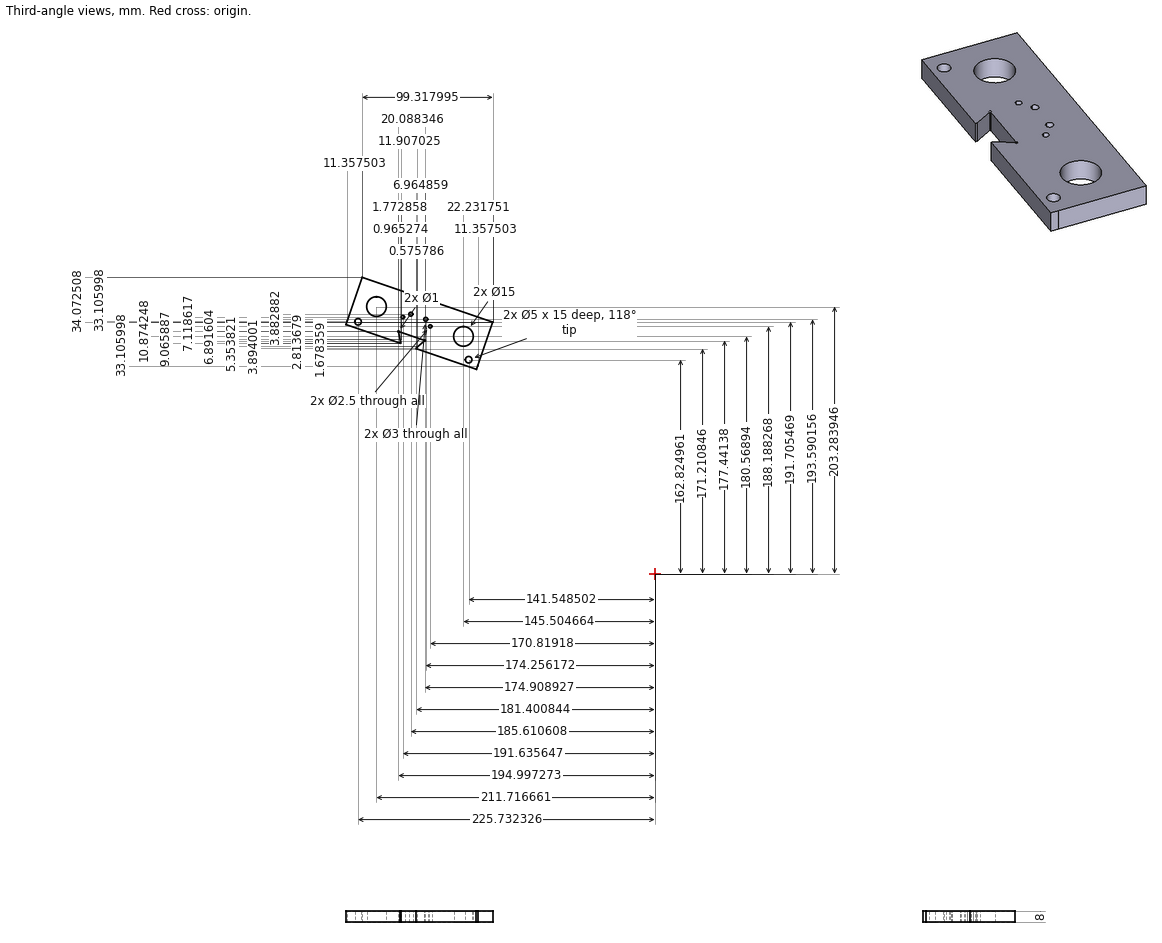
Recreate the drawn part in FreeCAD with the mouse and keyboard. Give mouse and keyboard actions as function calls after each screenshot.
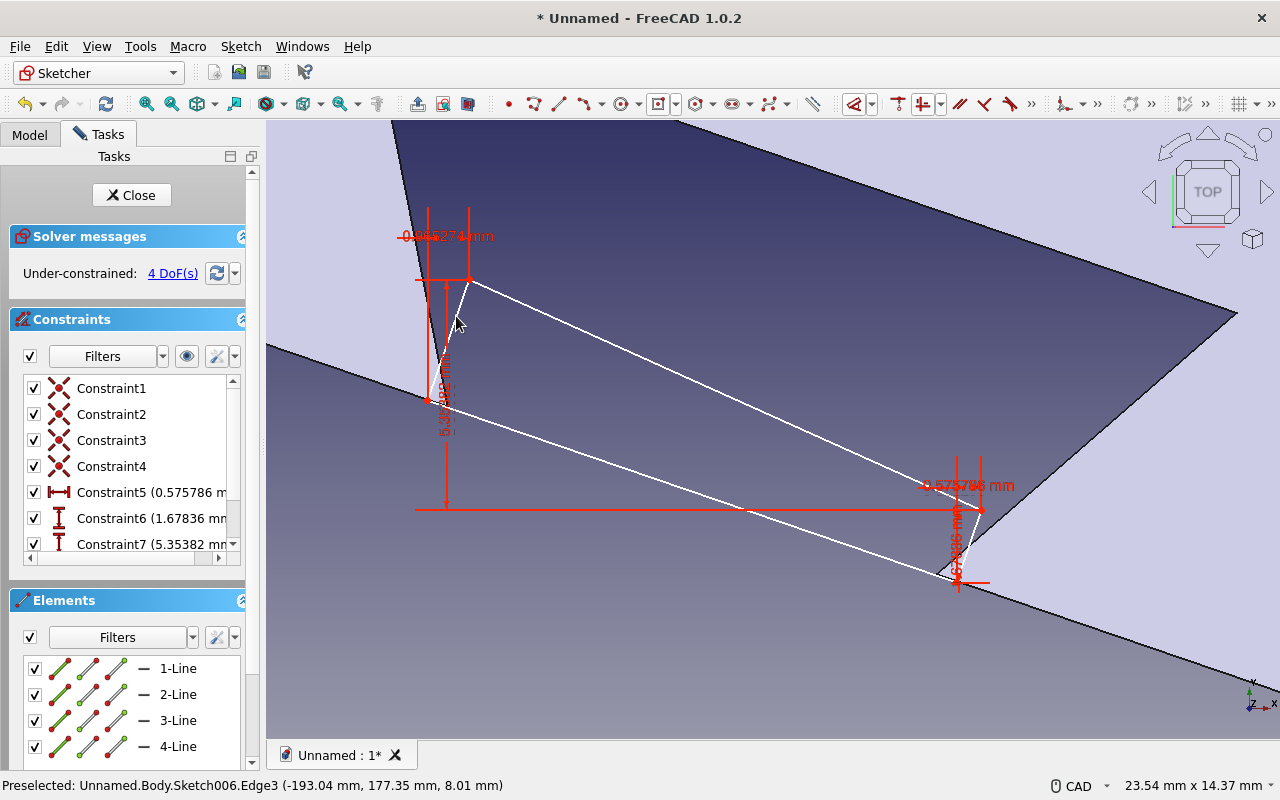
click(457, 316)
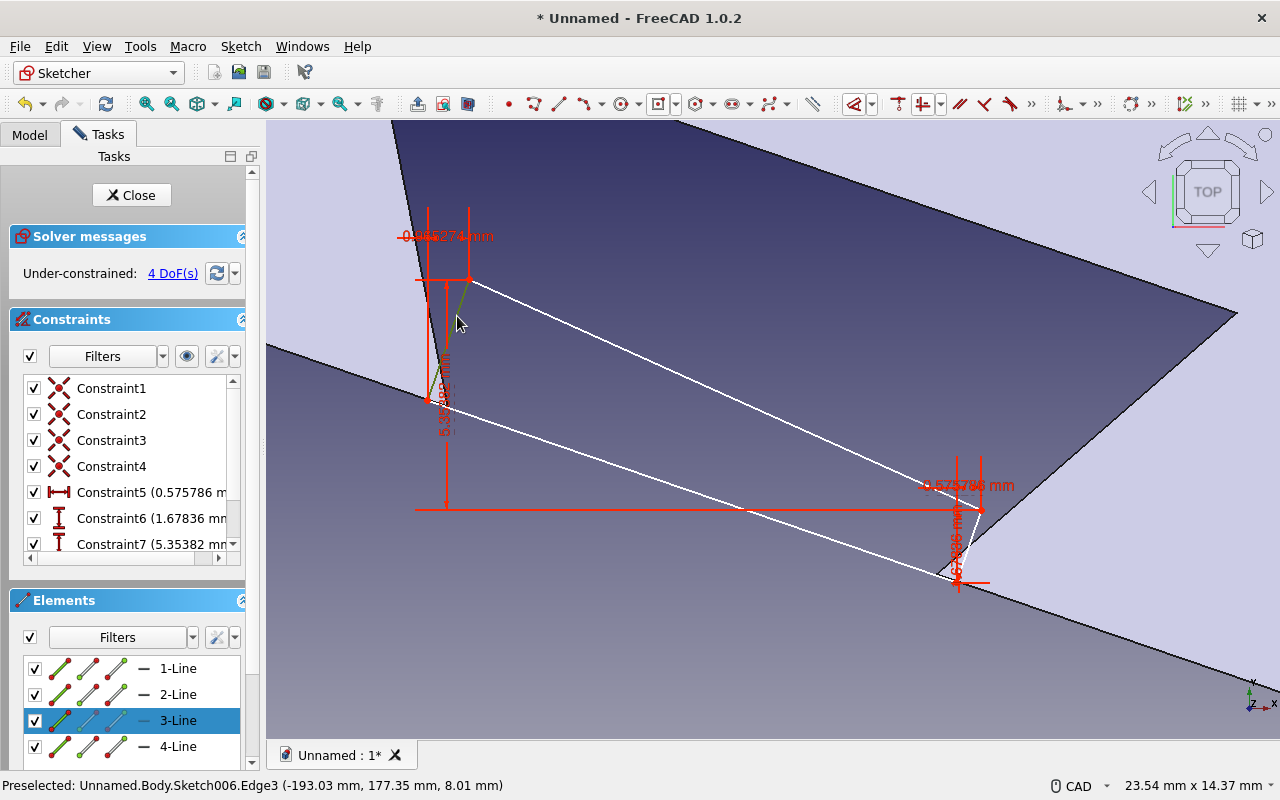
click(872, 104)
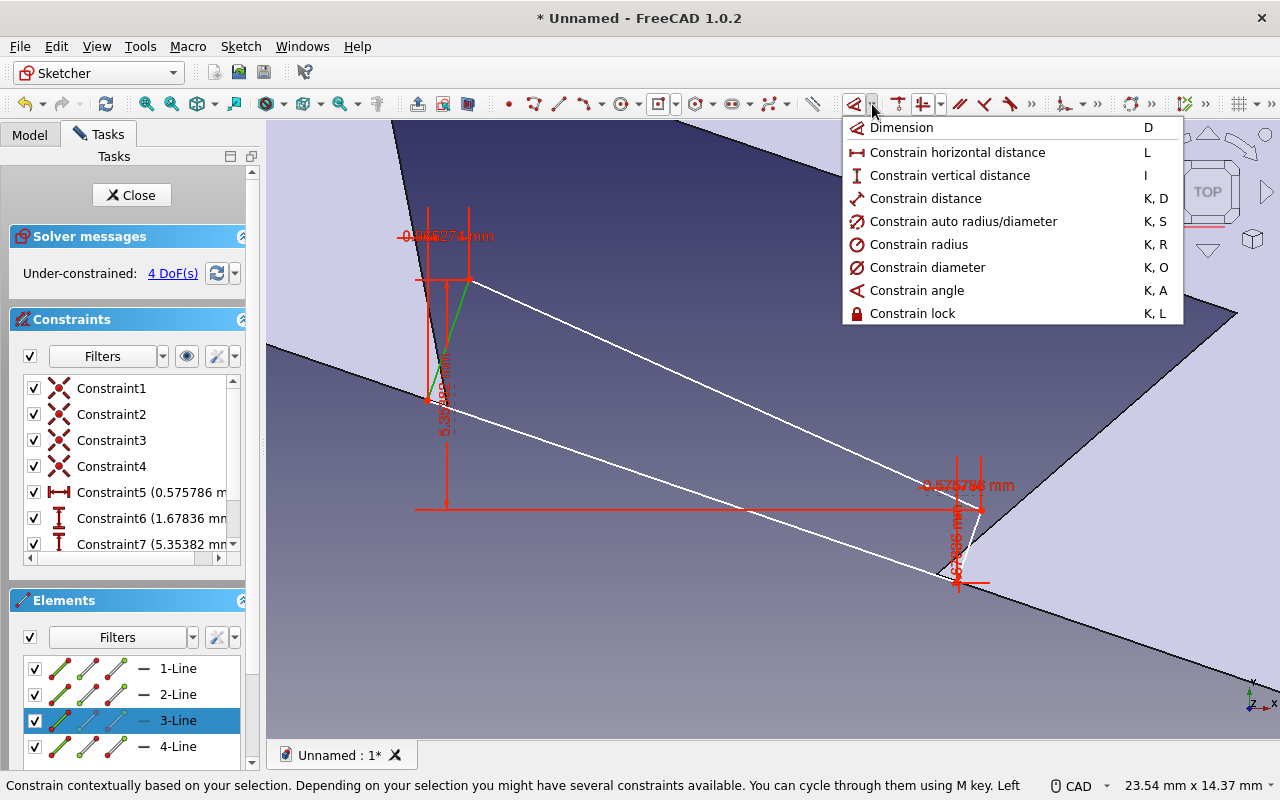
click(1013, 176)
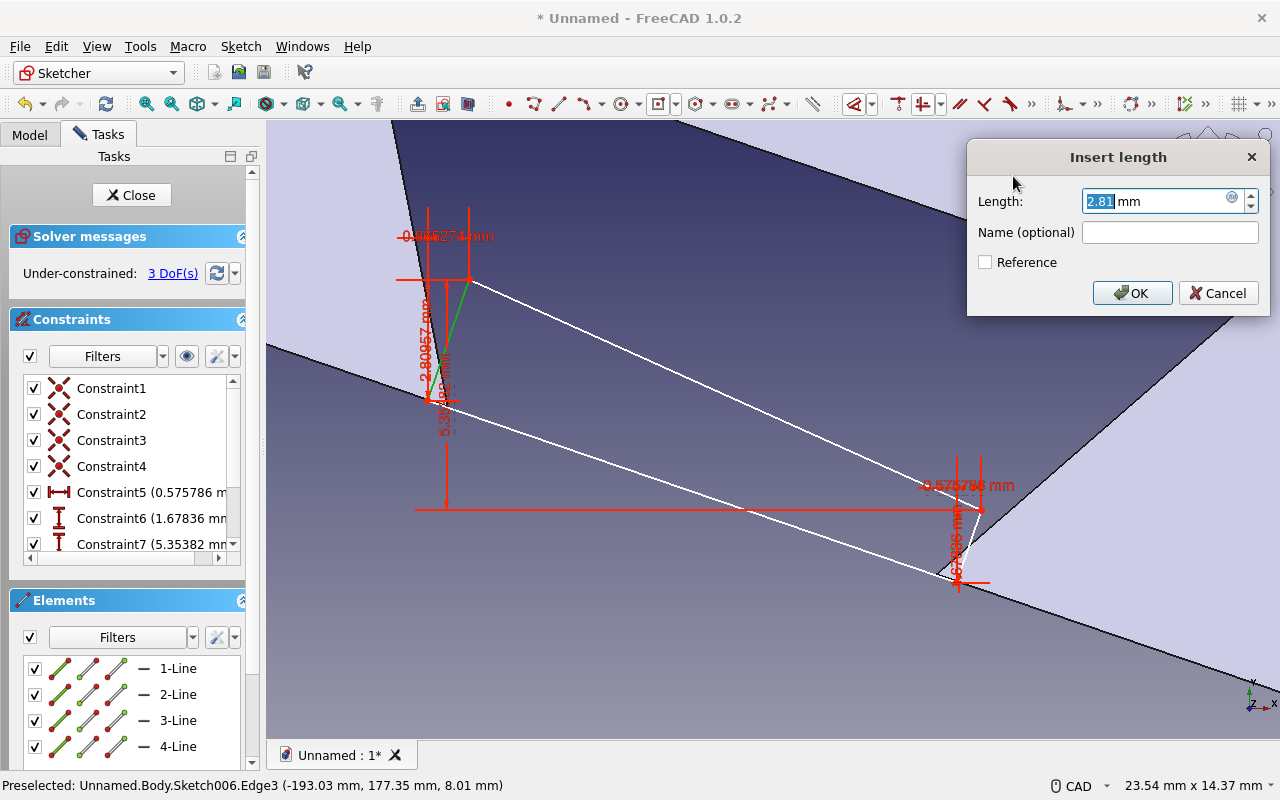
text(2.813679)
key(Return)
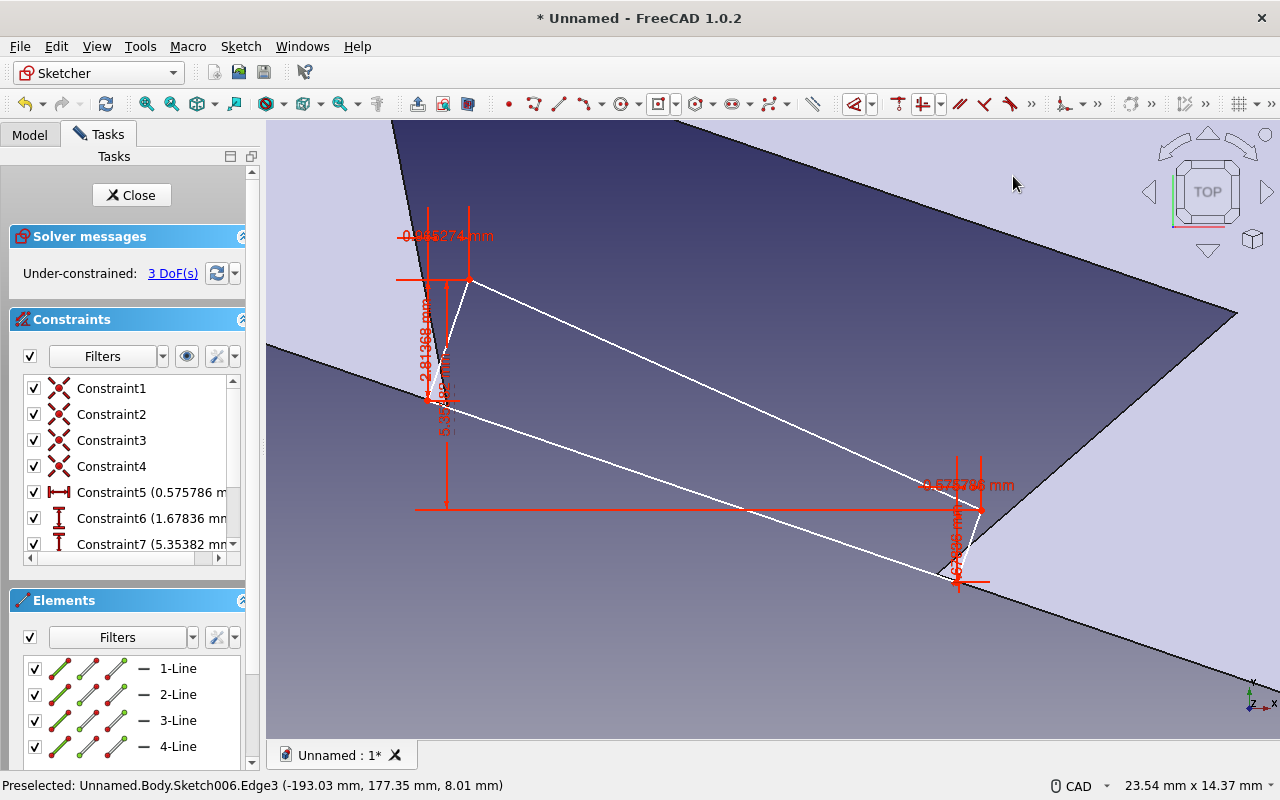
click(828, 441)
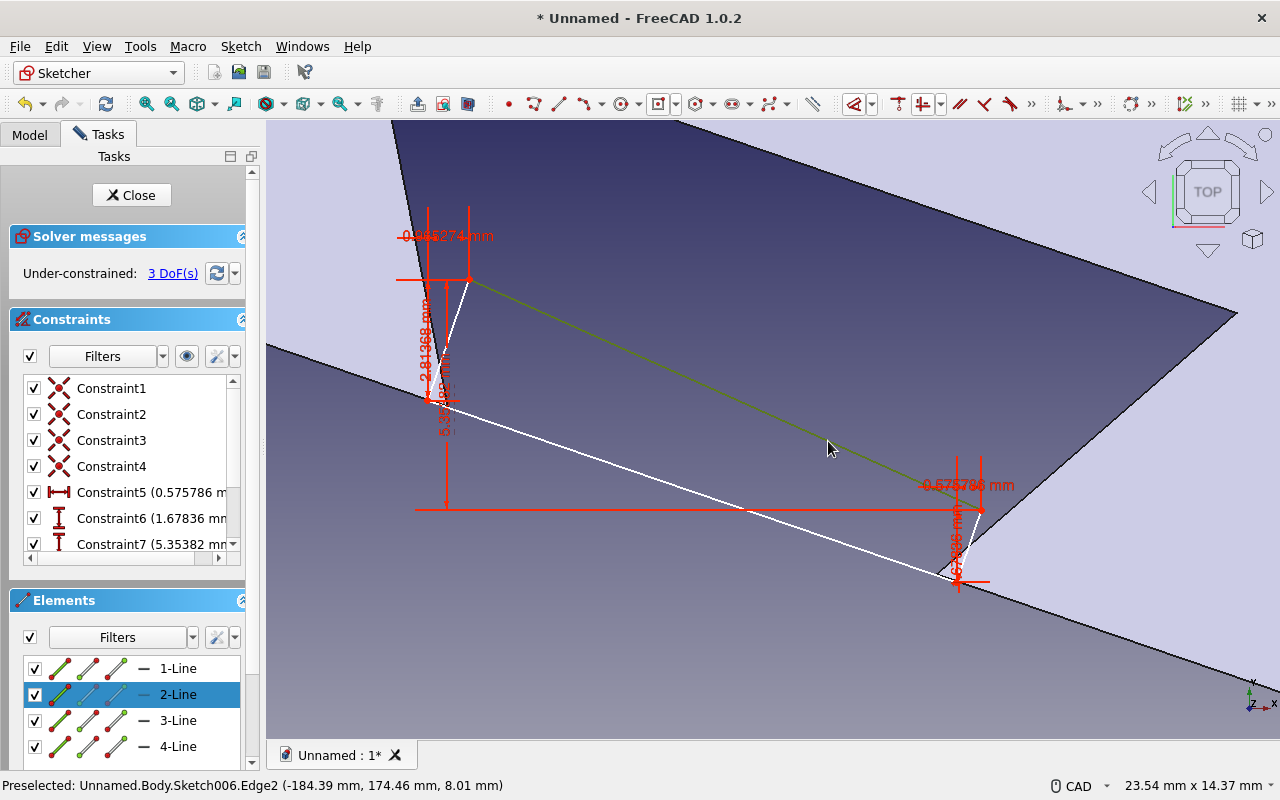
click(872, 104)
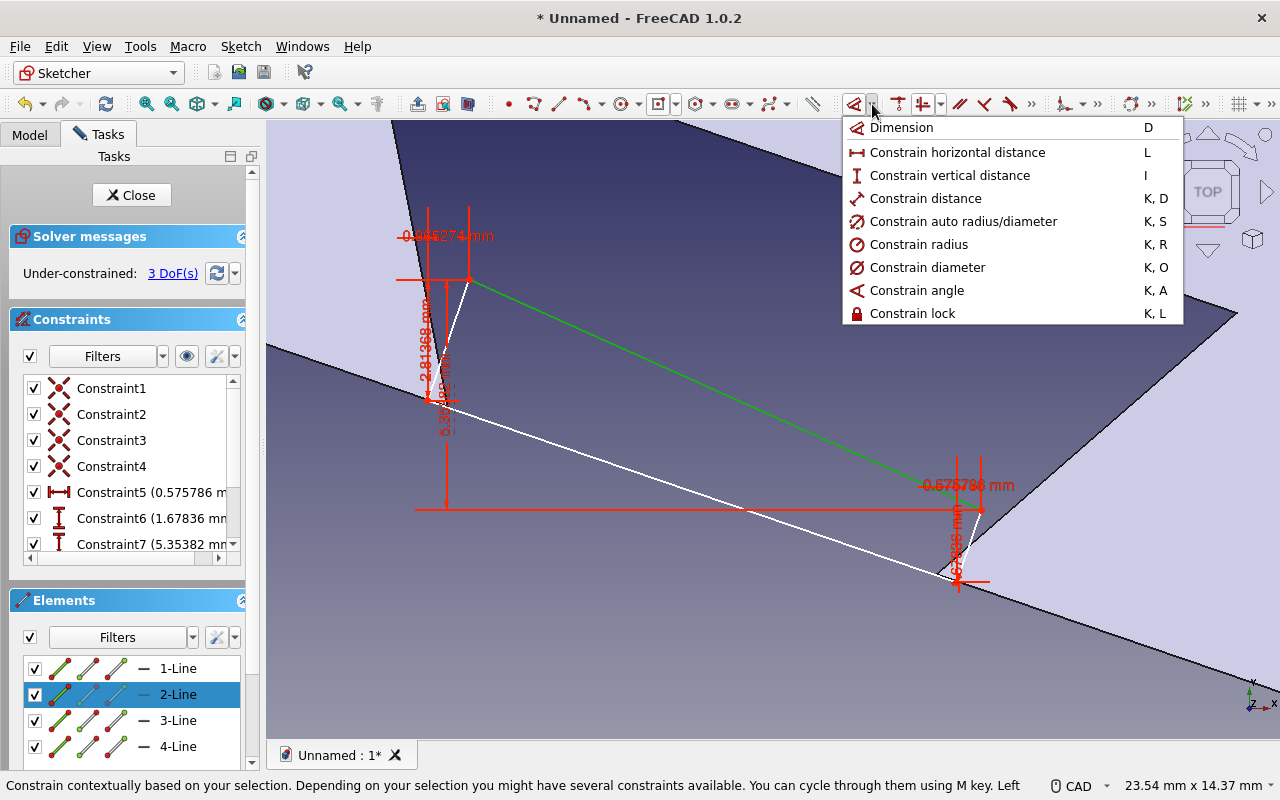
click(1013, 152)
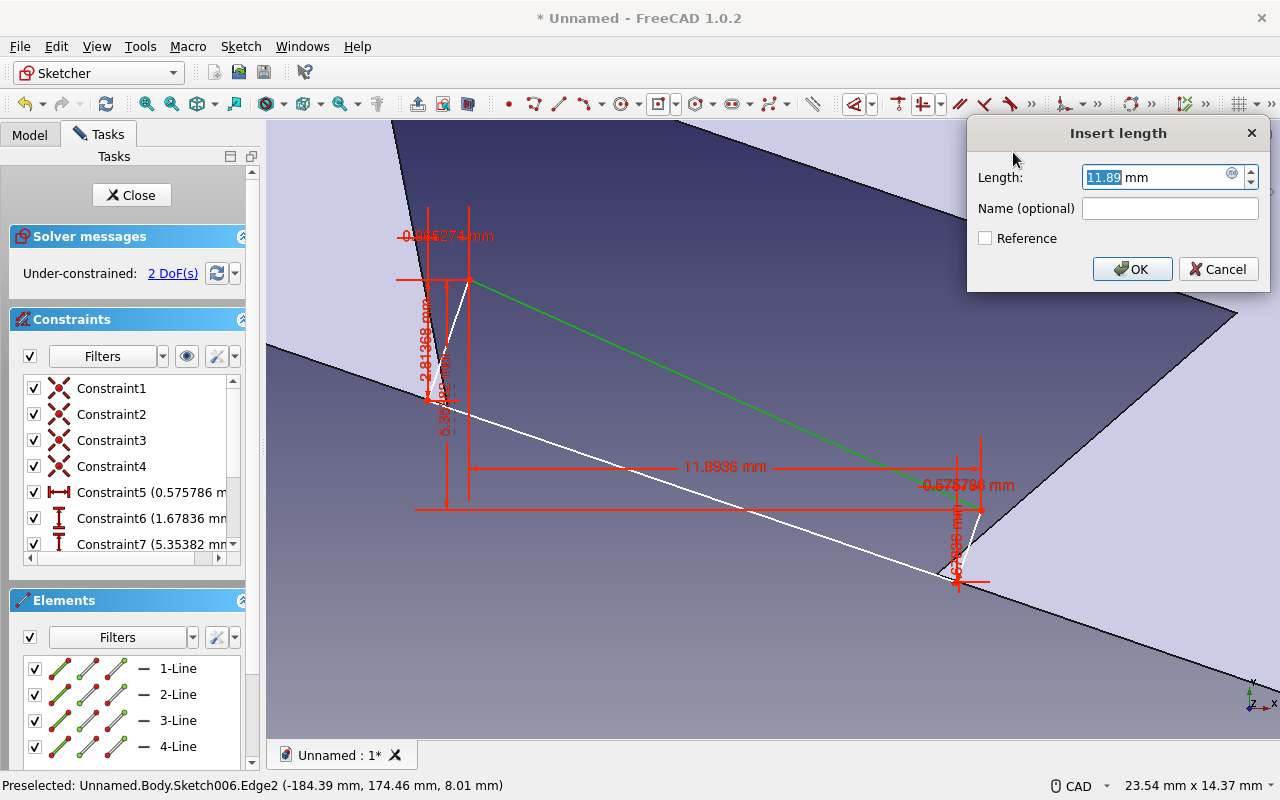
text(11.907025)
key(Return)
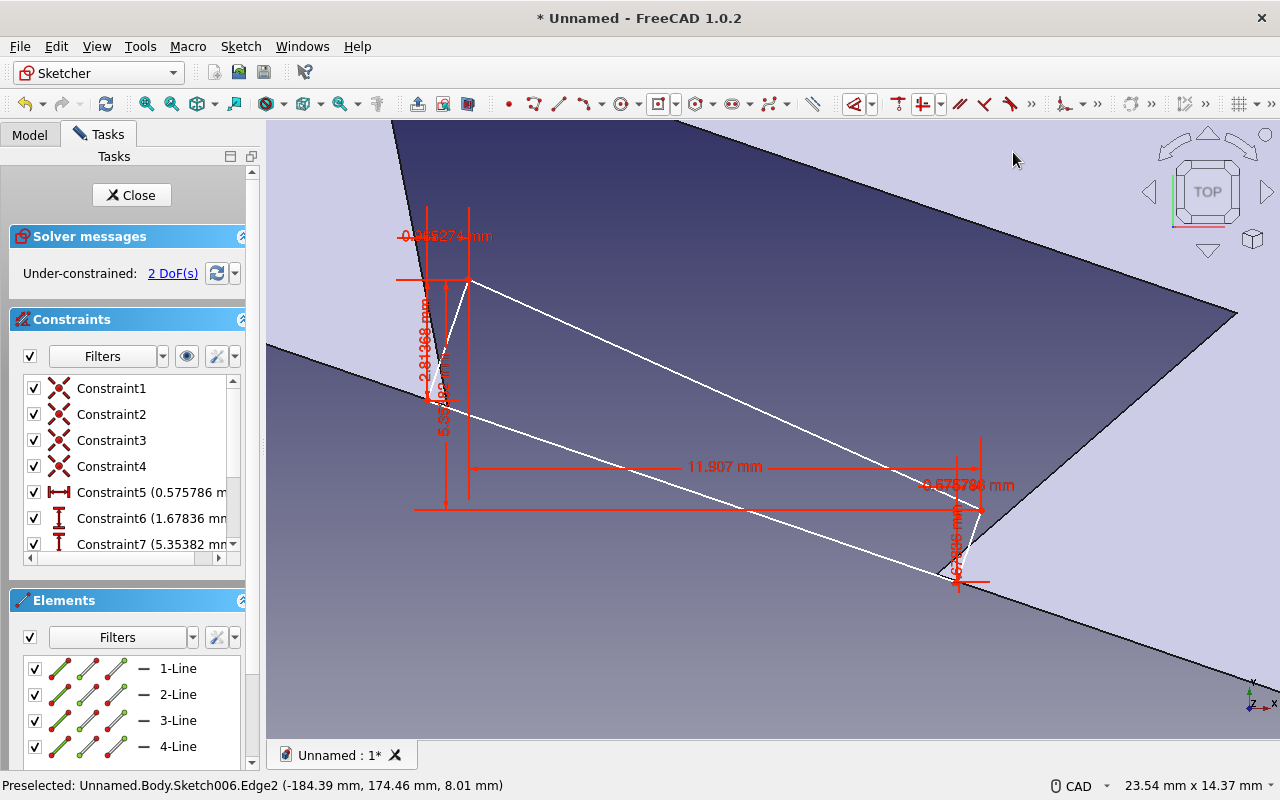
click(957, 582)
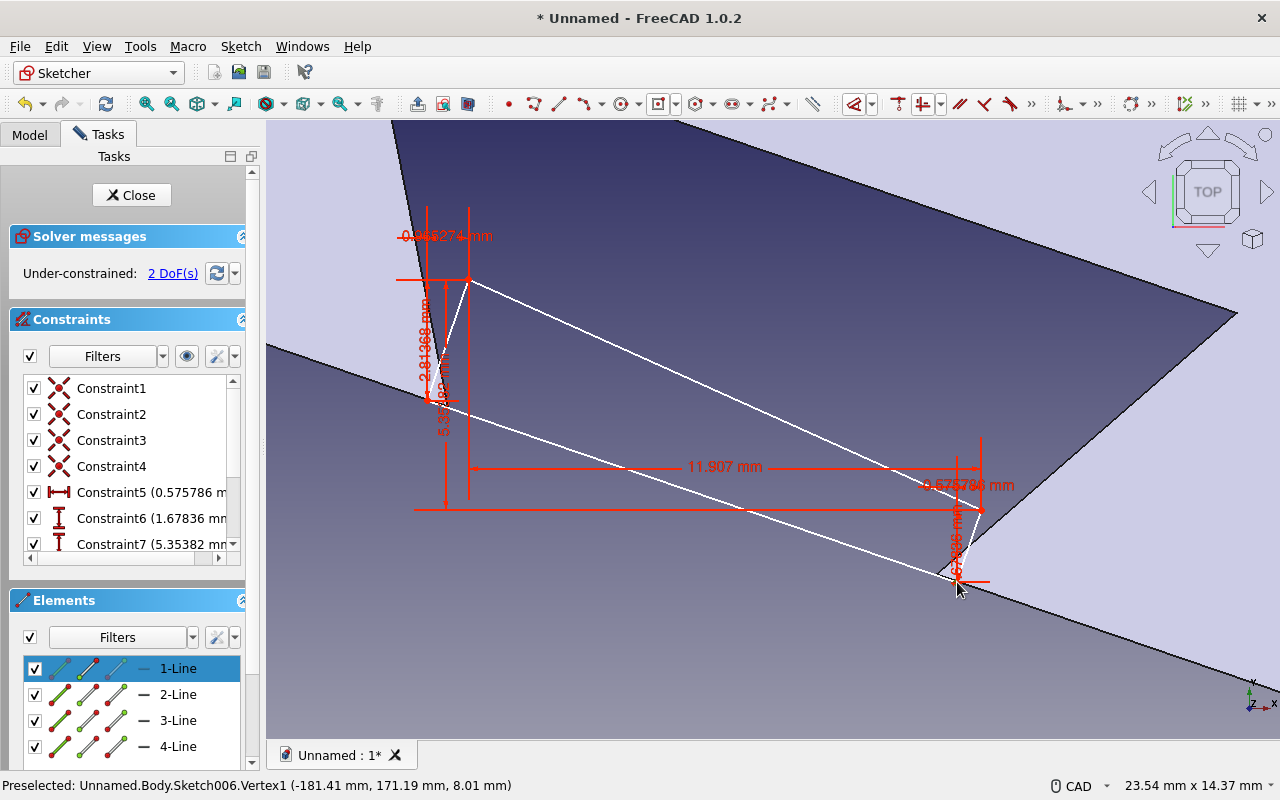
click(872, 104)